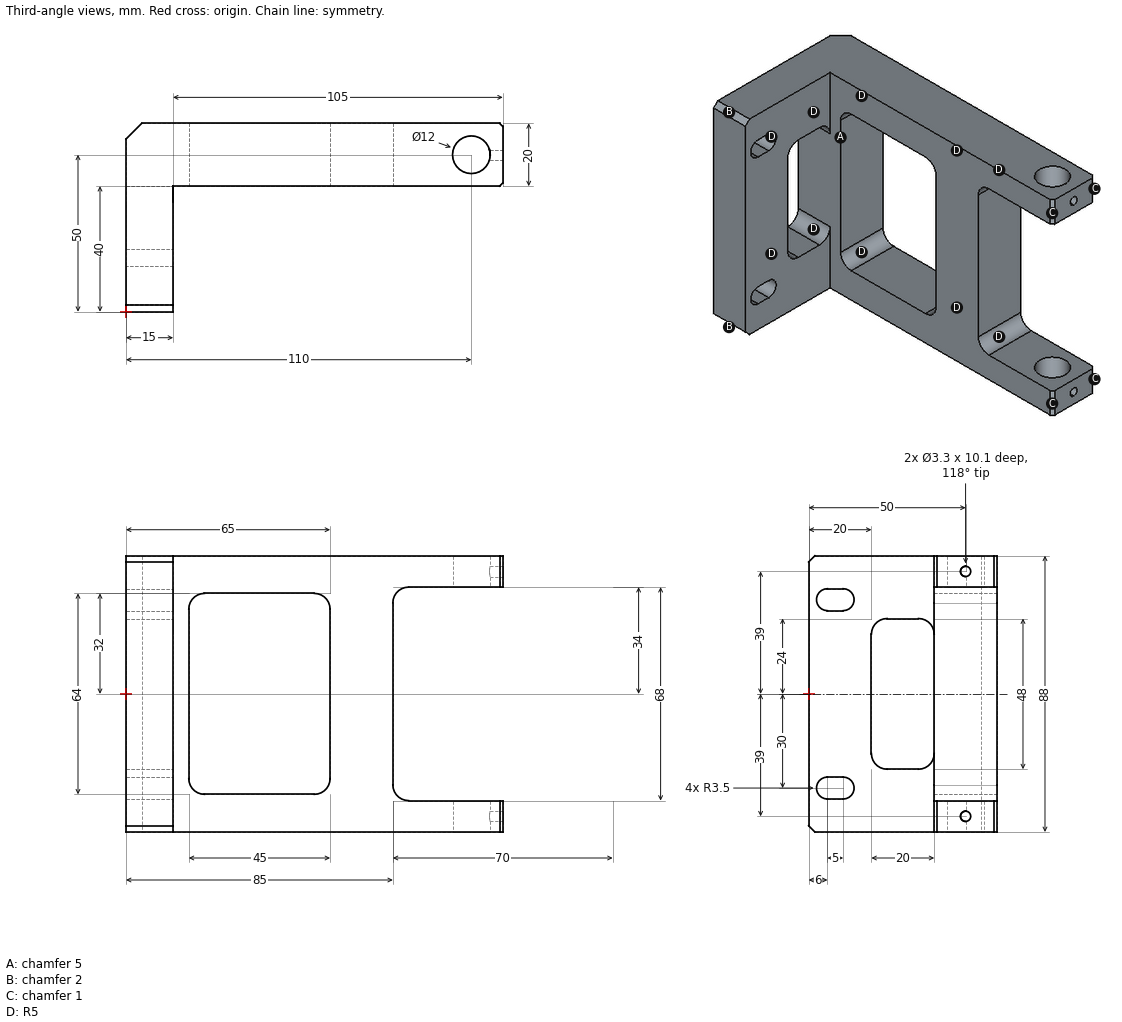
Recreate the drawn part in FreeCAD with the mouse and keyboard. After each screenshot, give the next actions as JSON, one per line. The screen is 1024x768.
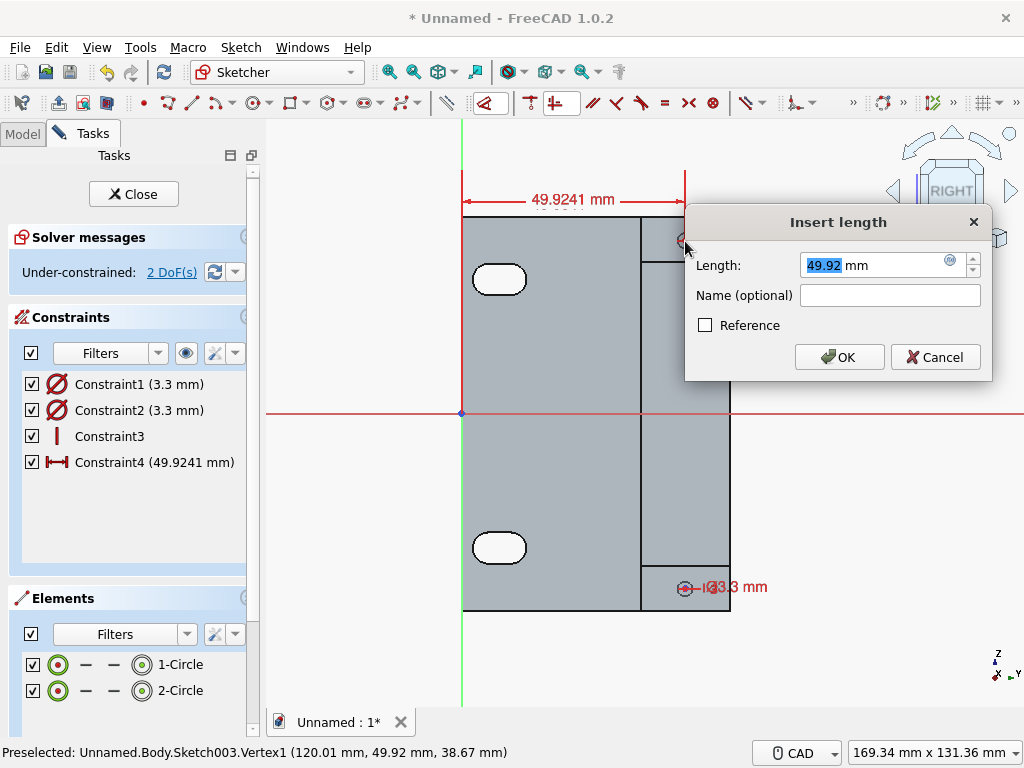
{"action": "type", "text": "50"}
{"action": "key", "text": "Return"}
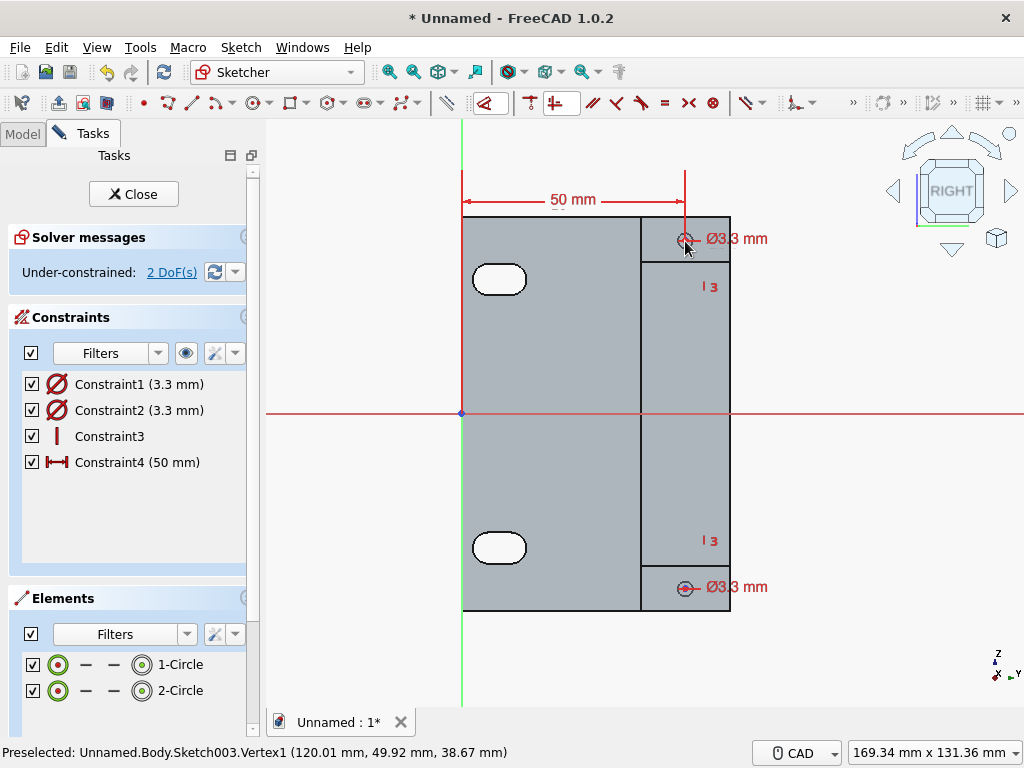
{"action": "left_click", "coordinate": [685, 241]}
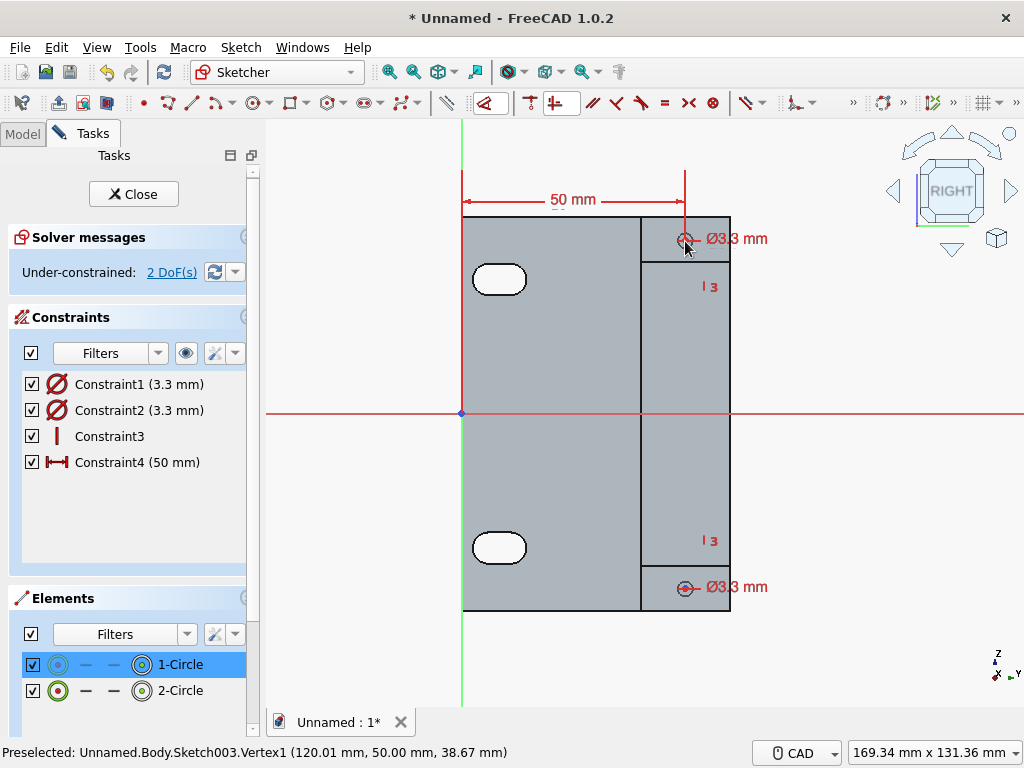
{"action": "key", "text": "i"}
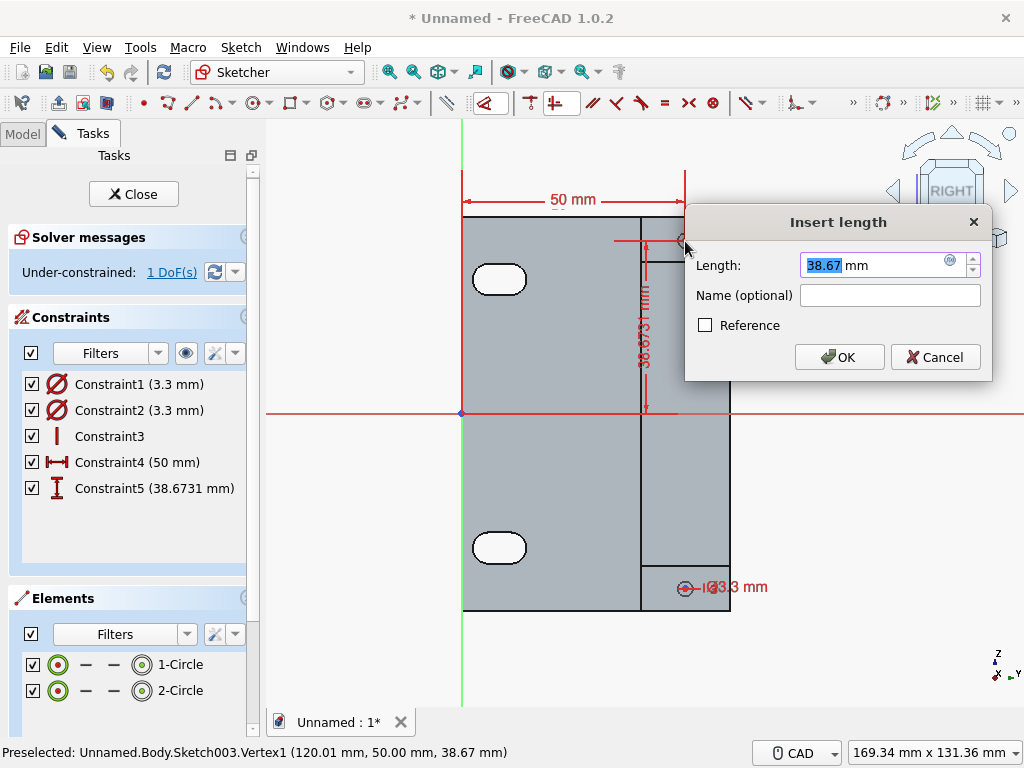
{"action": "type", "text": "39"}
{"action": "key", "text": "Return"}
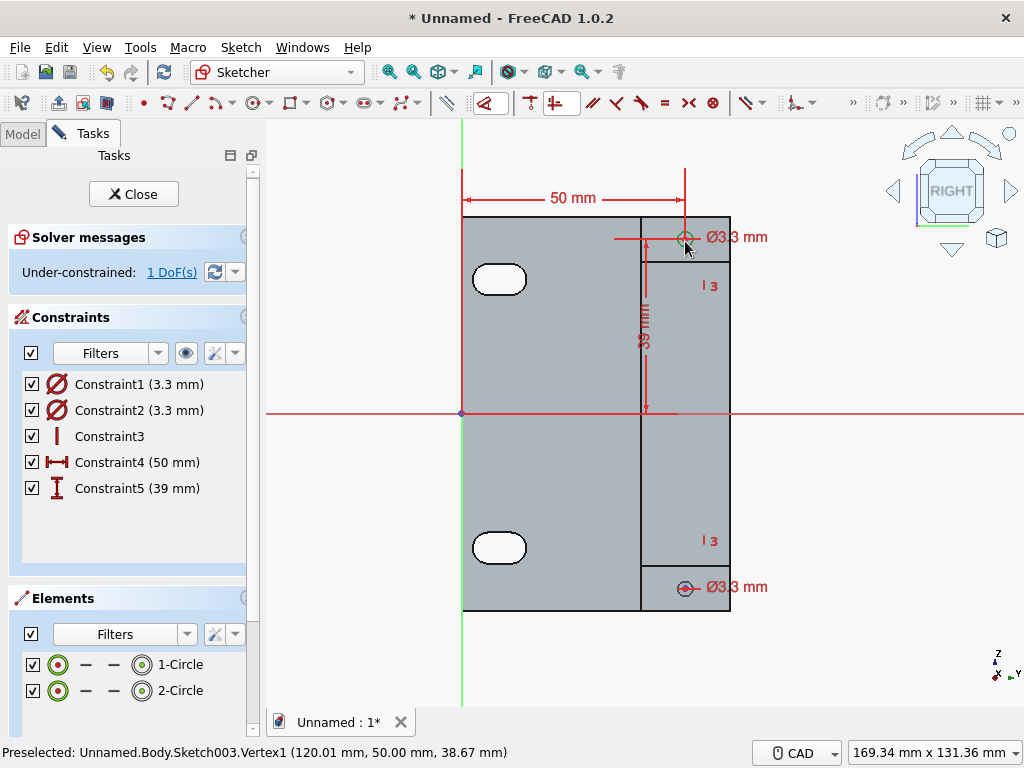
{"action": "left_click", "coordinate": [685, 589]}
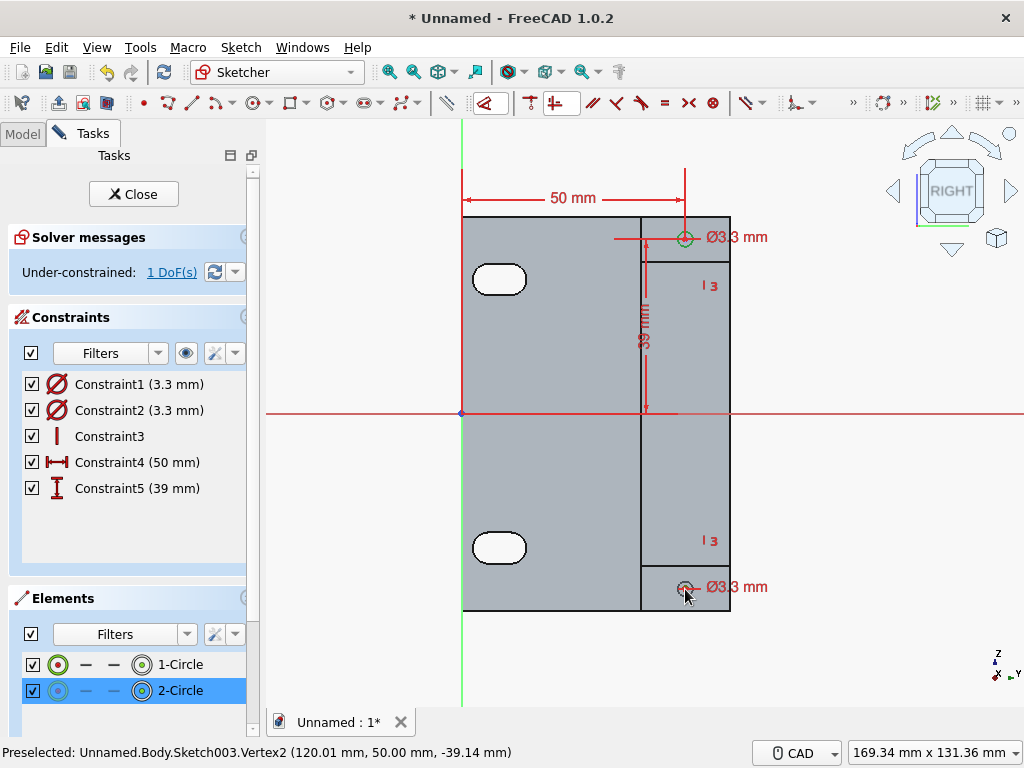
{"action": "key", "text": "i"}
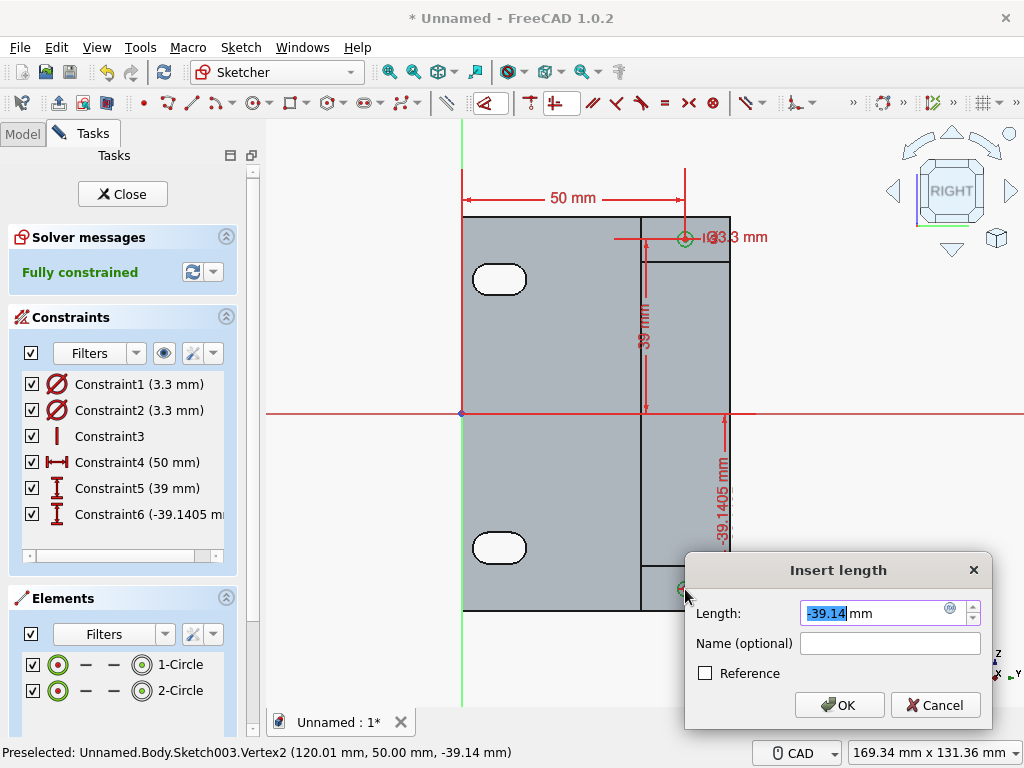
{"action": "type", "text": "-39"}
{"action": "key", "text": "Return"}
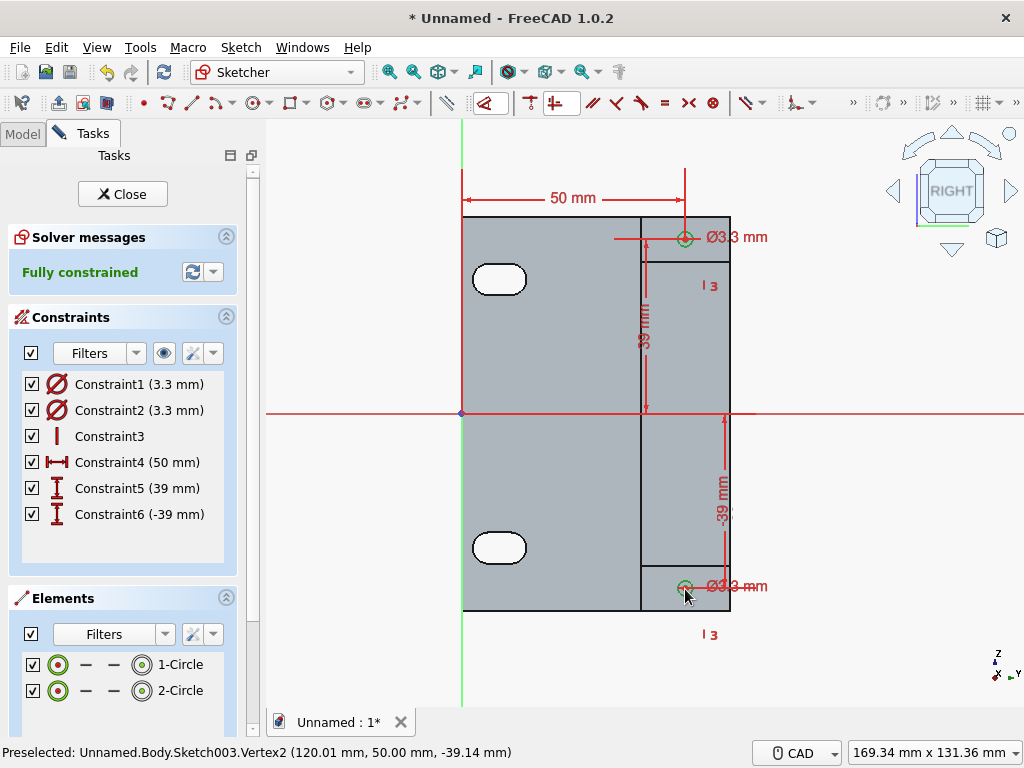
{"action": "left_click", "coordinate": [123, 194]}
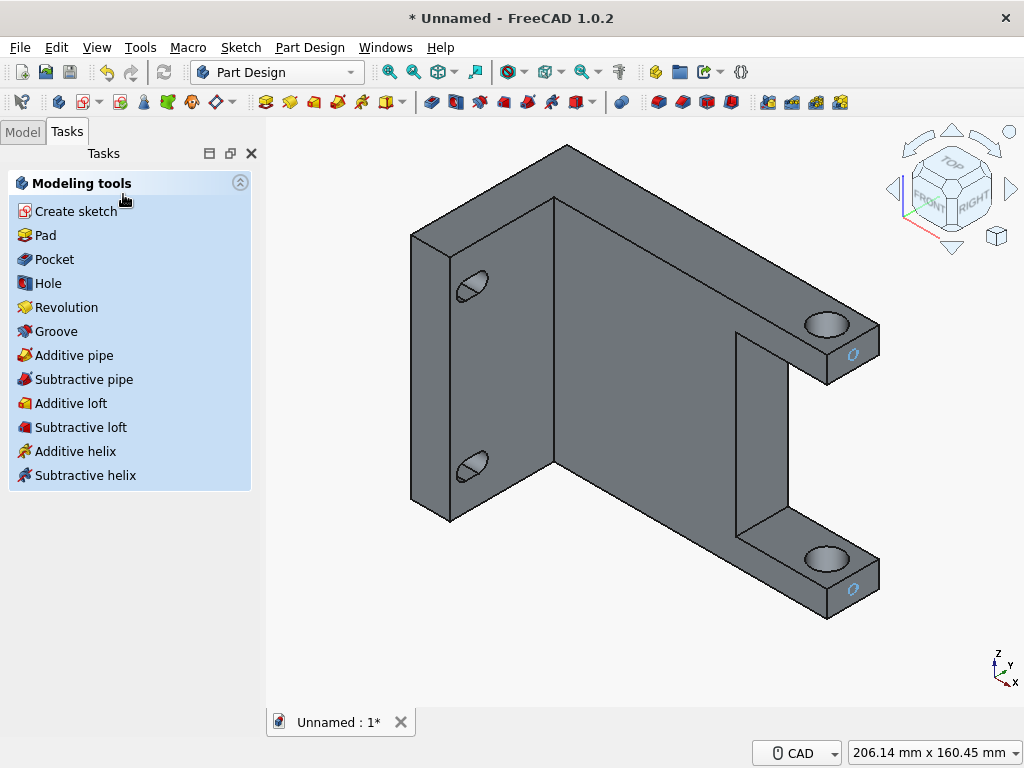
{"action": "left_click", "coordinate": [456, 102]}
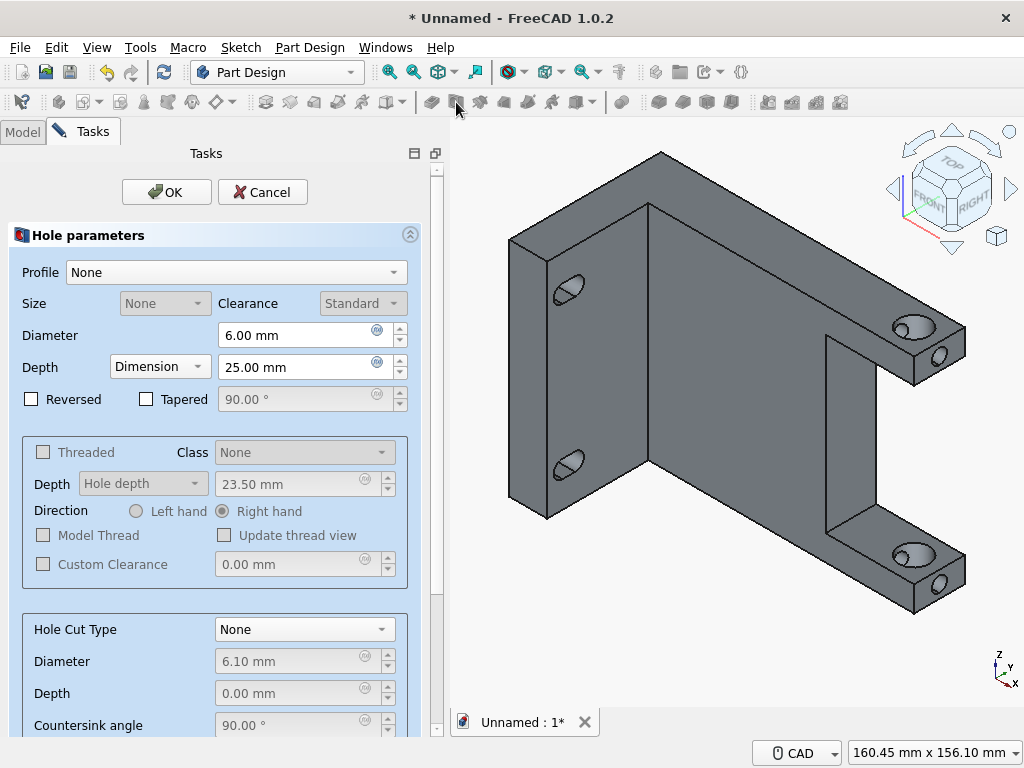
{"action": "triple_click", "coordinate": [305, 335]}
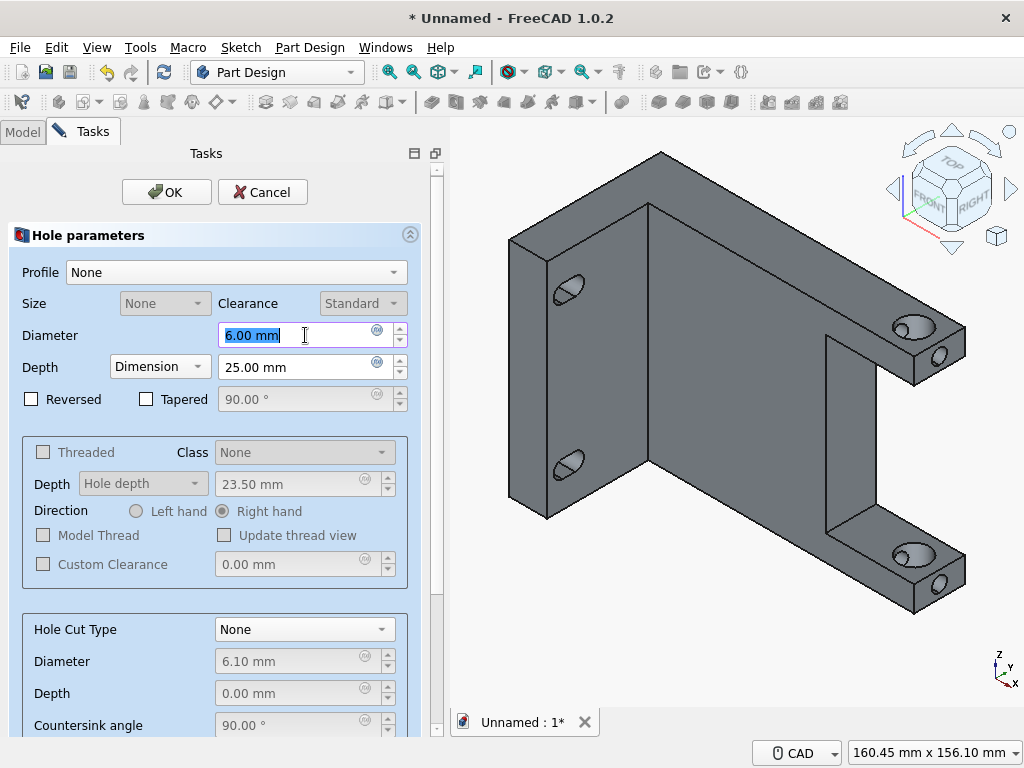
{"action": "type", "text": "3.3"}
{"action": "key", "text": "Tab"}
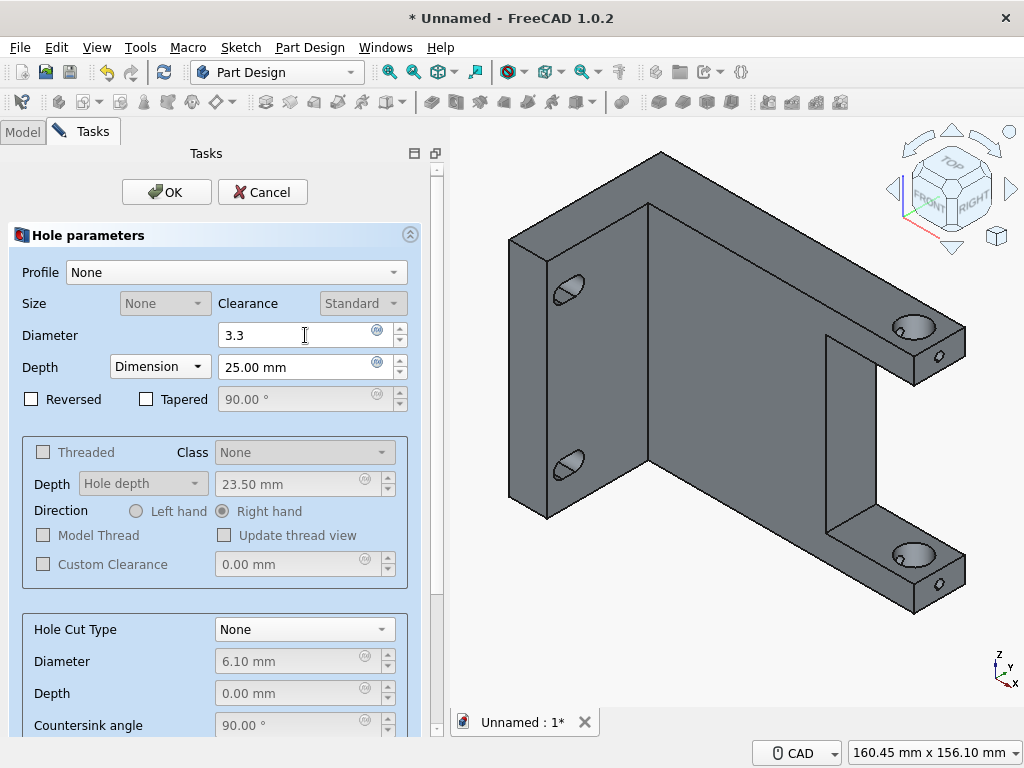
{"action": "triple_click", "coordinate": [305, 367]}